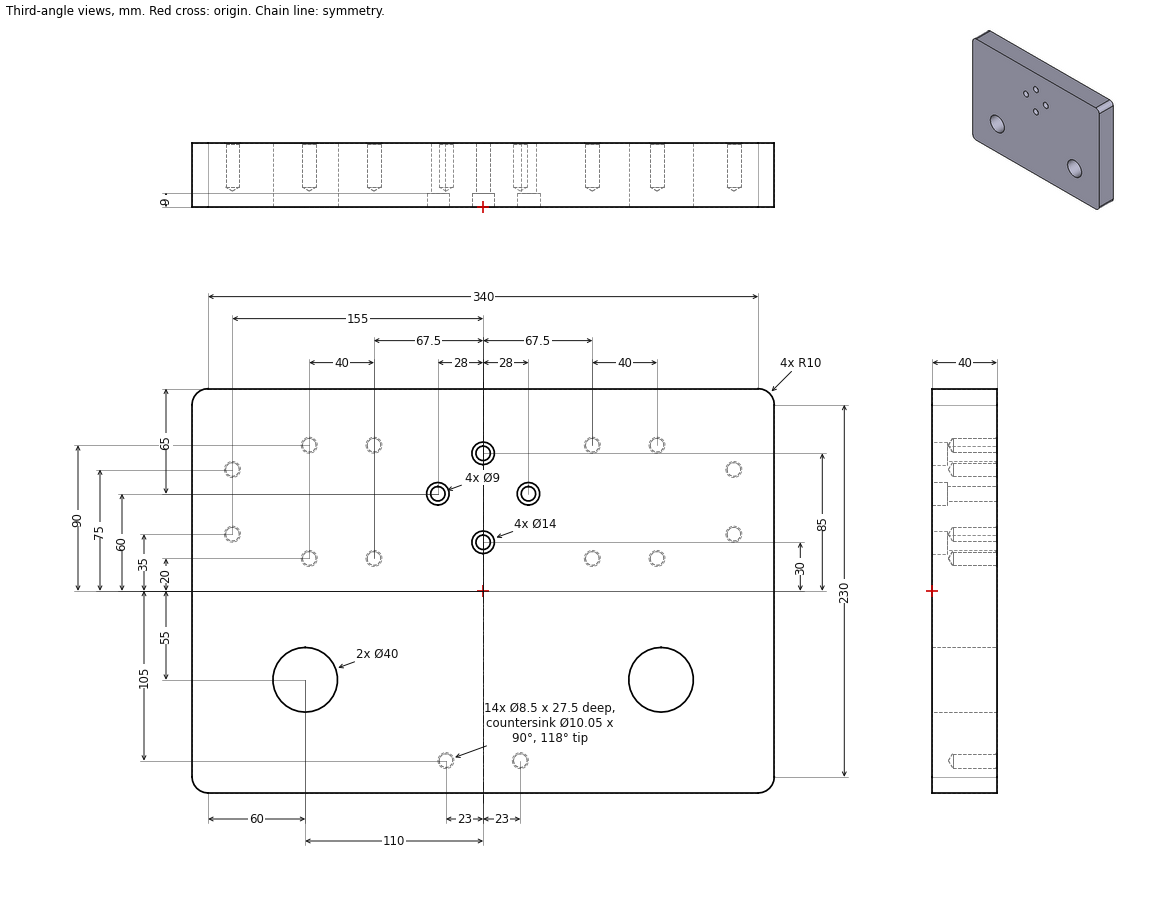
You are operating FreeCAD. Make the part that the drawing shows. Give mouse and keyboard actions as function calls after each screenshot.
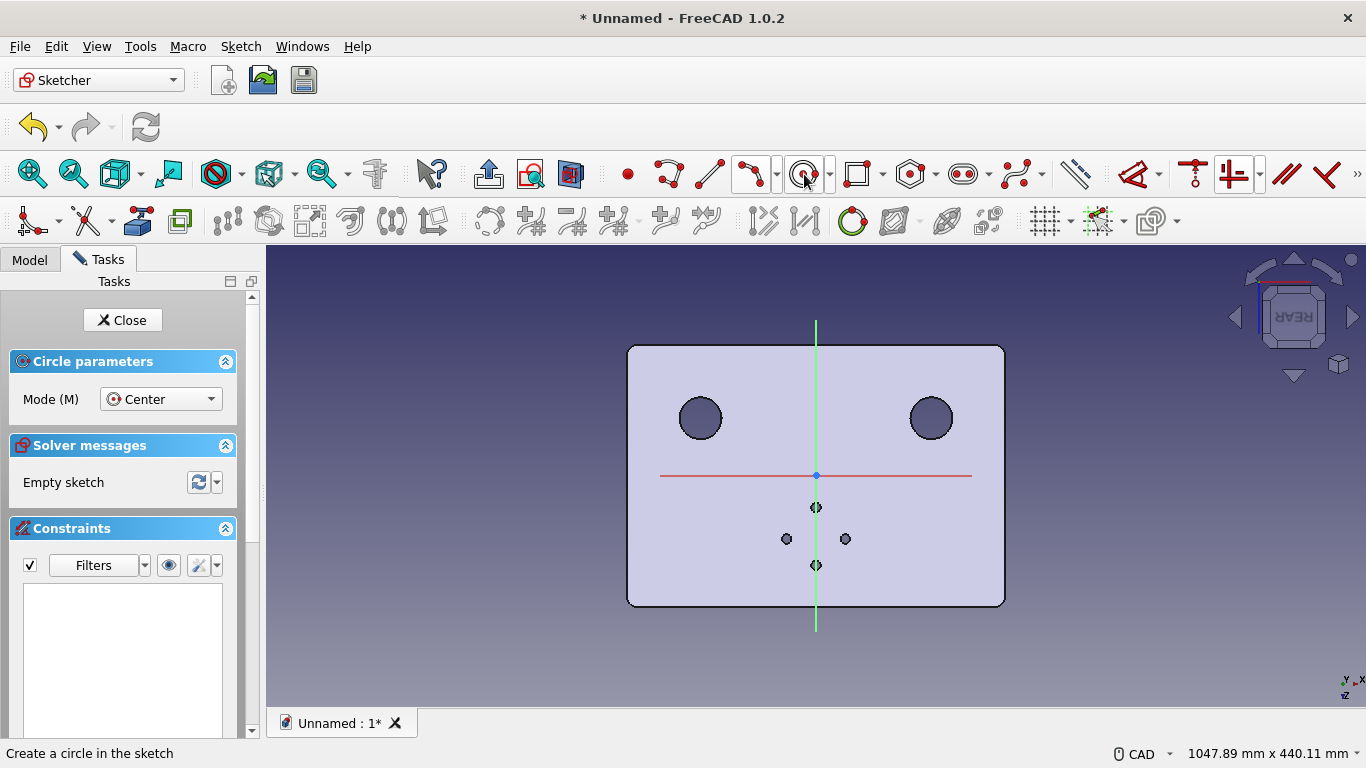
scroll(792, 366, up, 9)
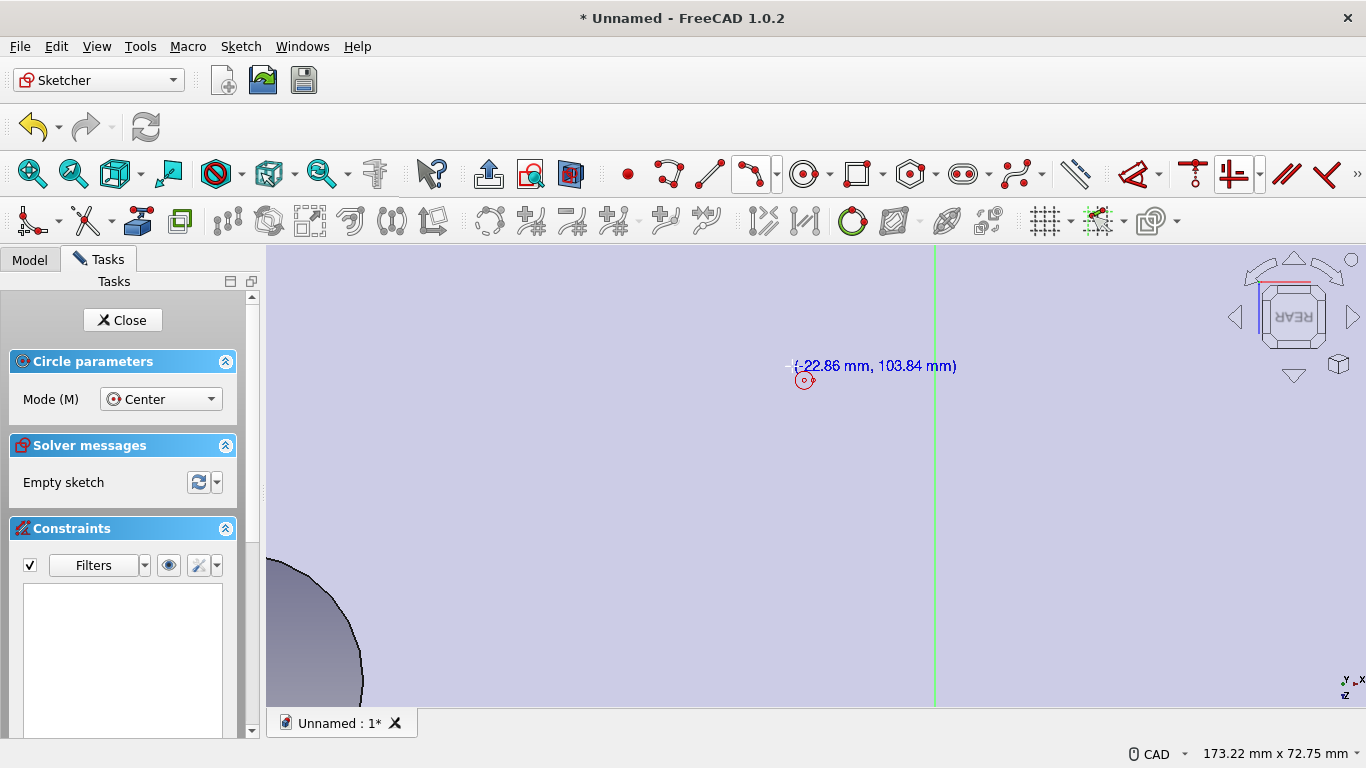
scroll(700, 348, down, 8)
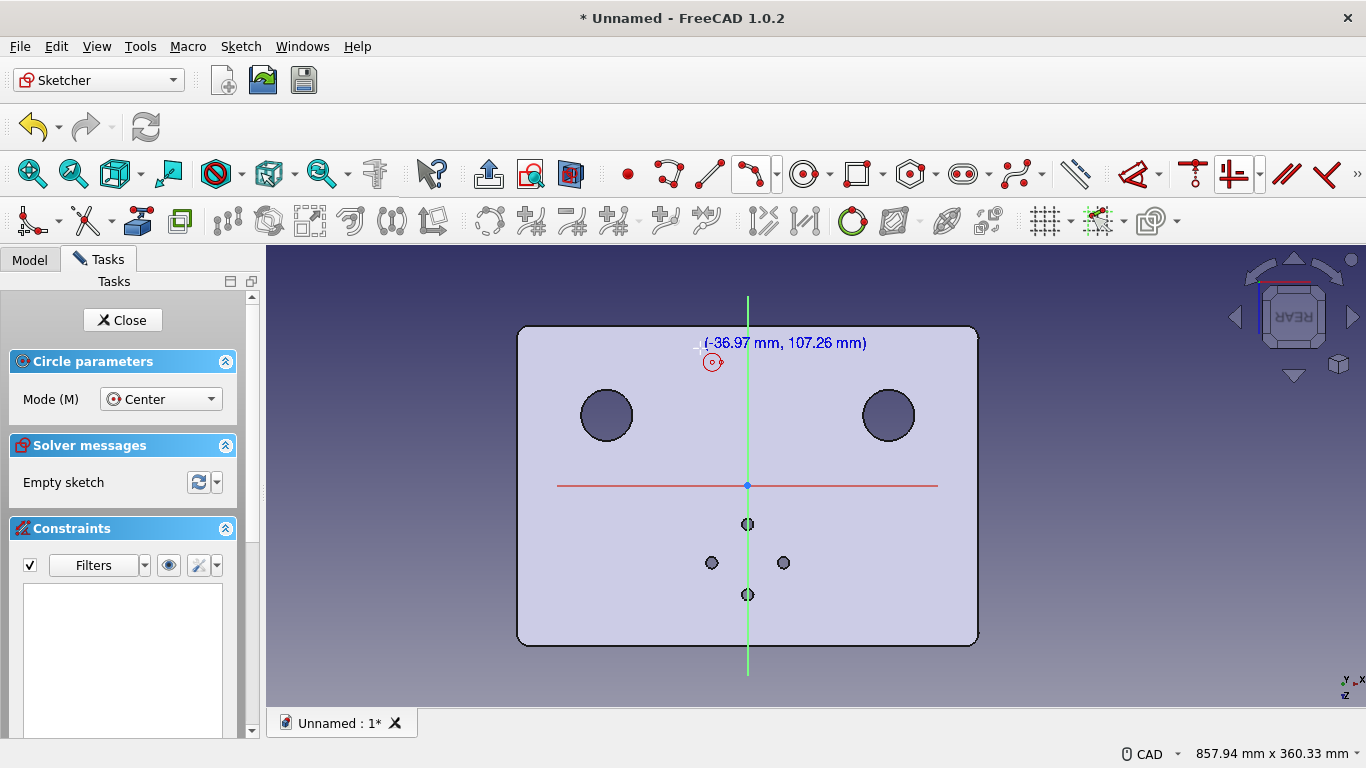
click(718, 351)
move(722, 347)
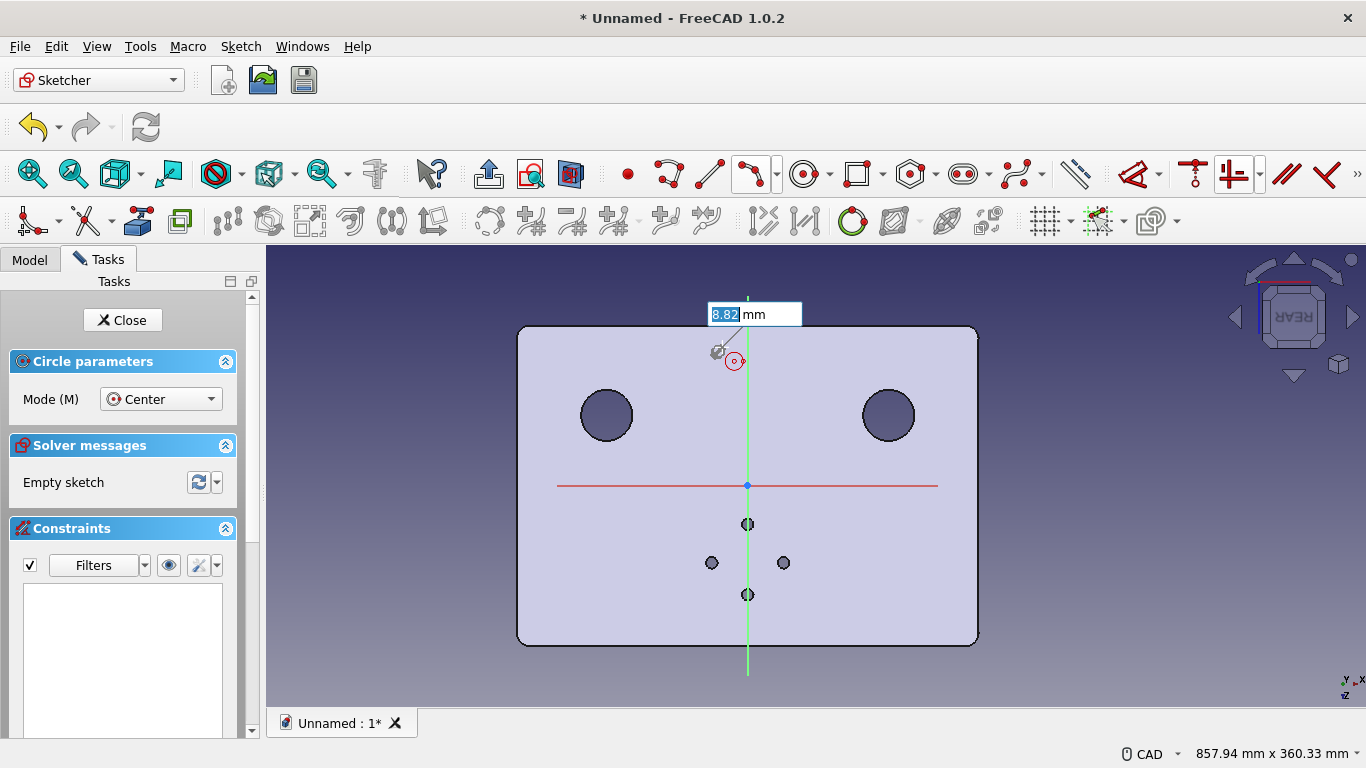
text(8.5)
key(Return)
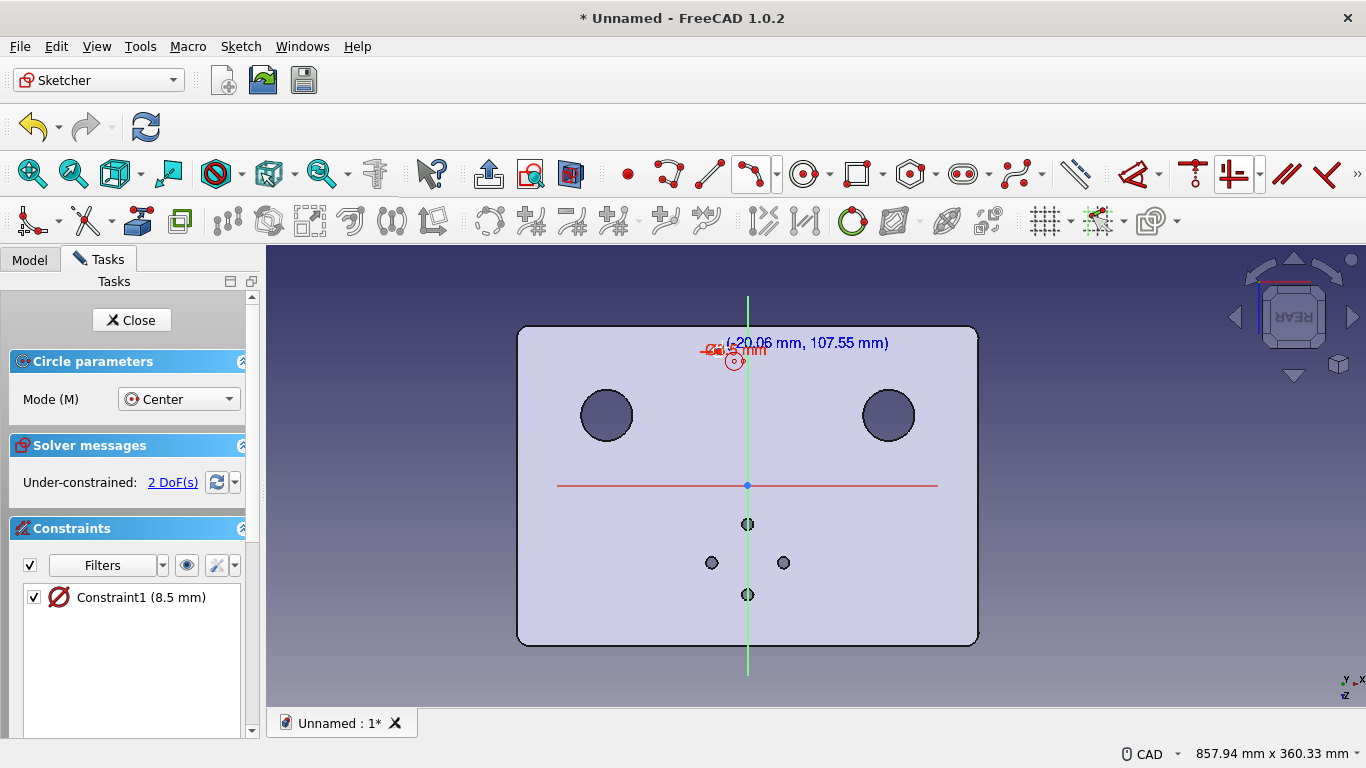
scroll(549, 531, up, 8)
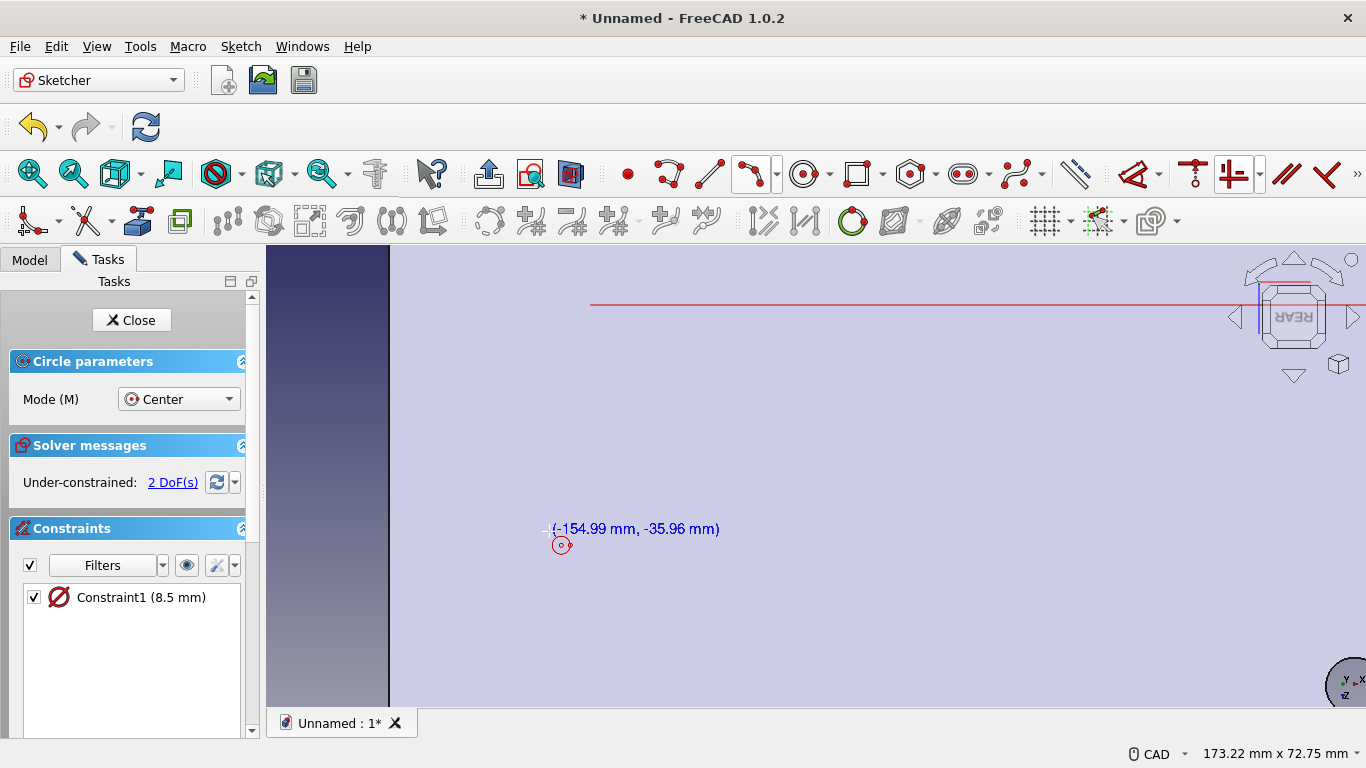
scroll(549, 531, down, 8)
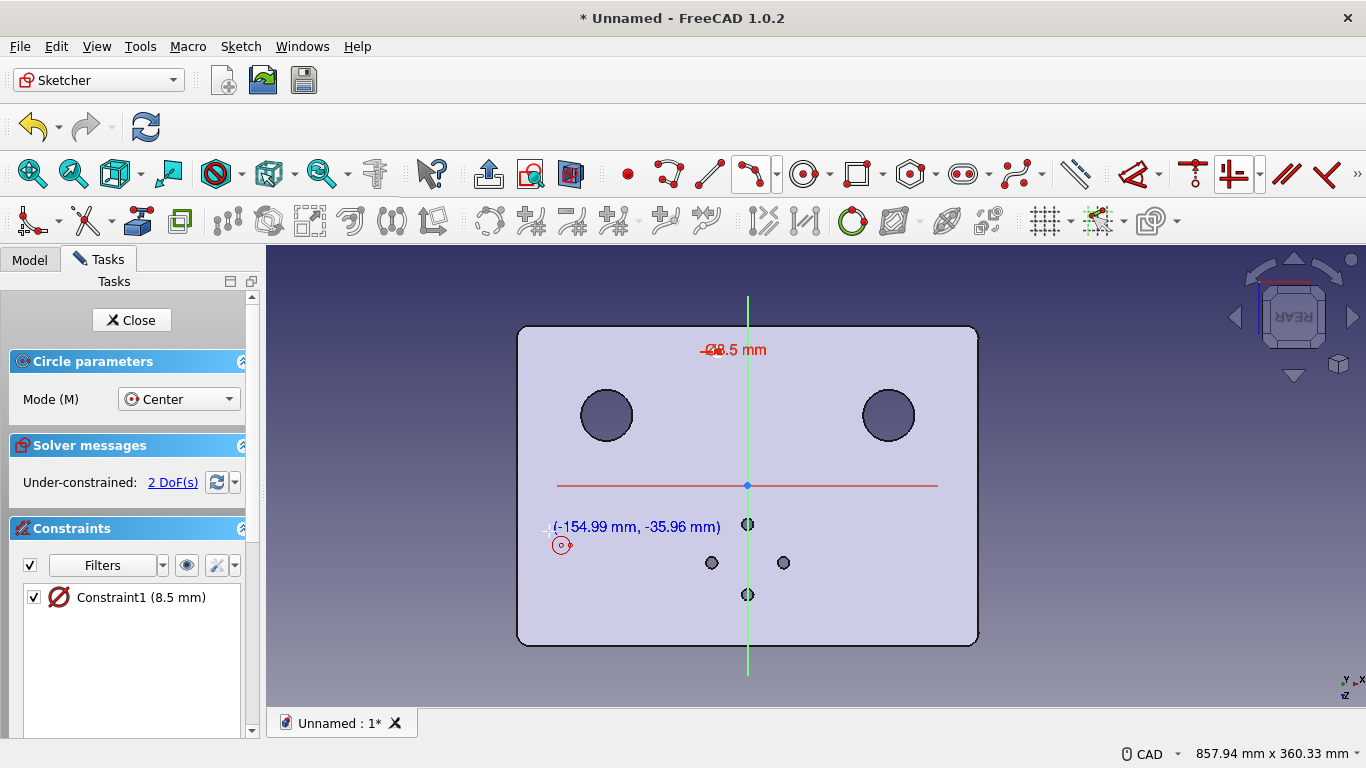
click(549, 531)
move(553, 527)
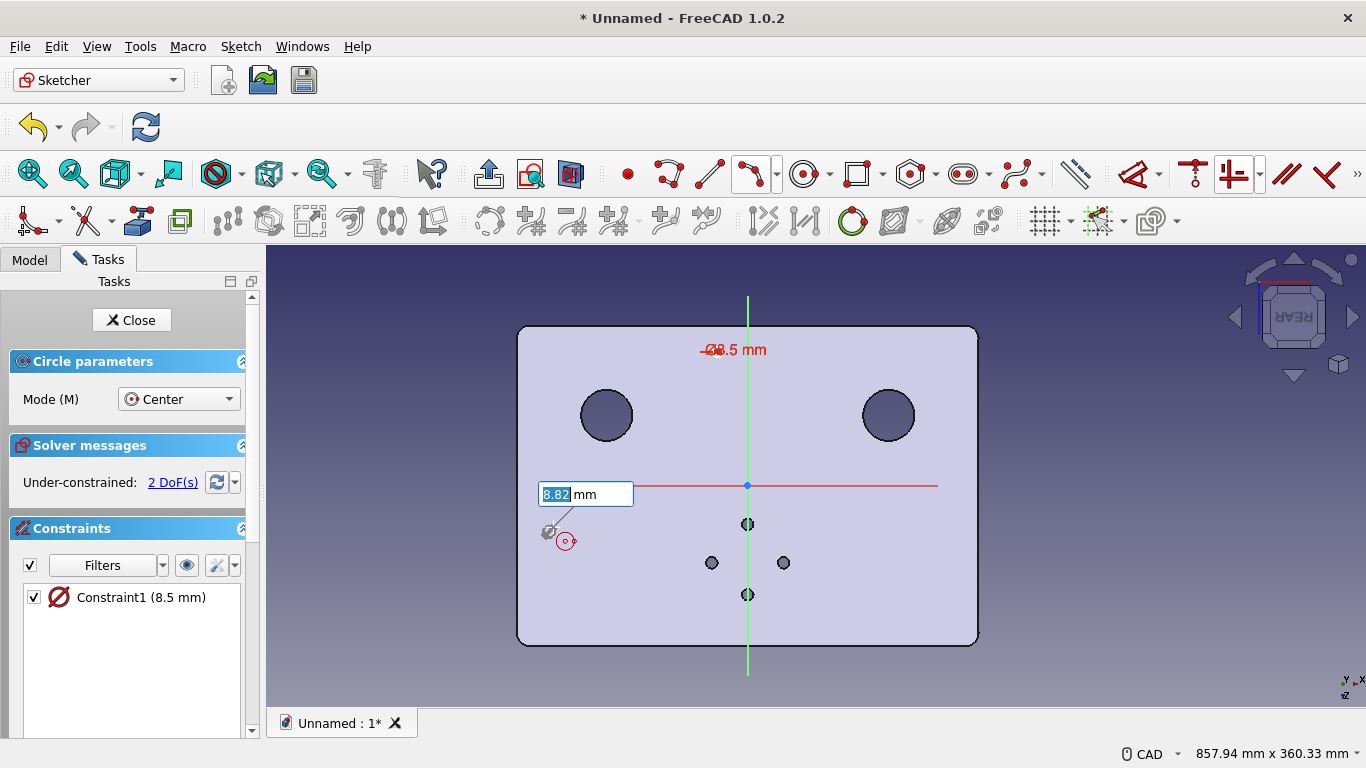
text(8.5)
key(Return)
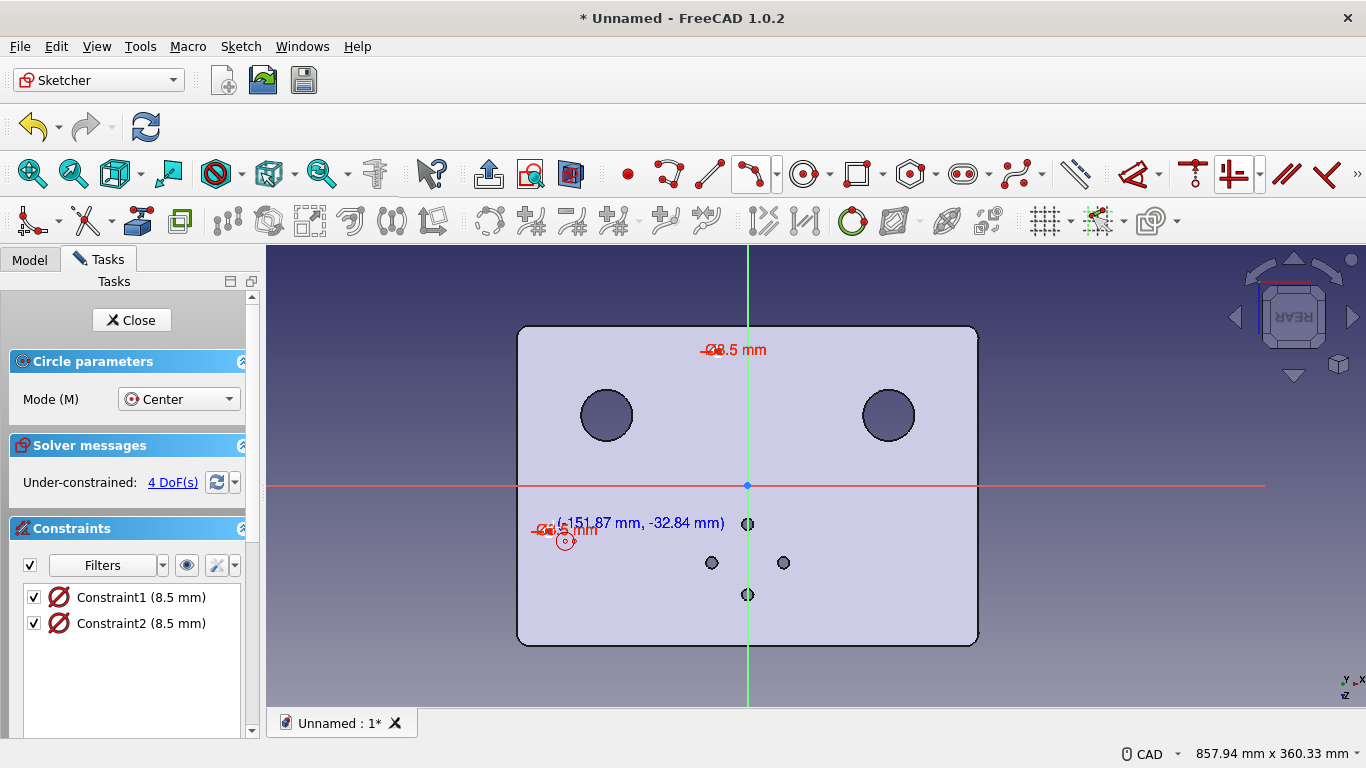
scroll(549, 582, up, 8)